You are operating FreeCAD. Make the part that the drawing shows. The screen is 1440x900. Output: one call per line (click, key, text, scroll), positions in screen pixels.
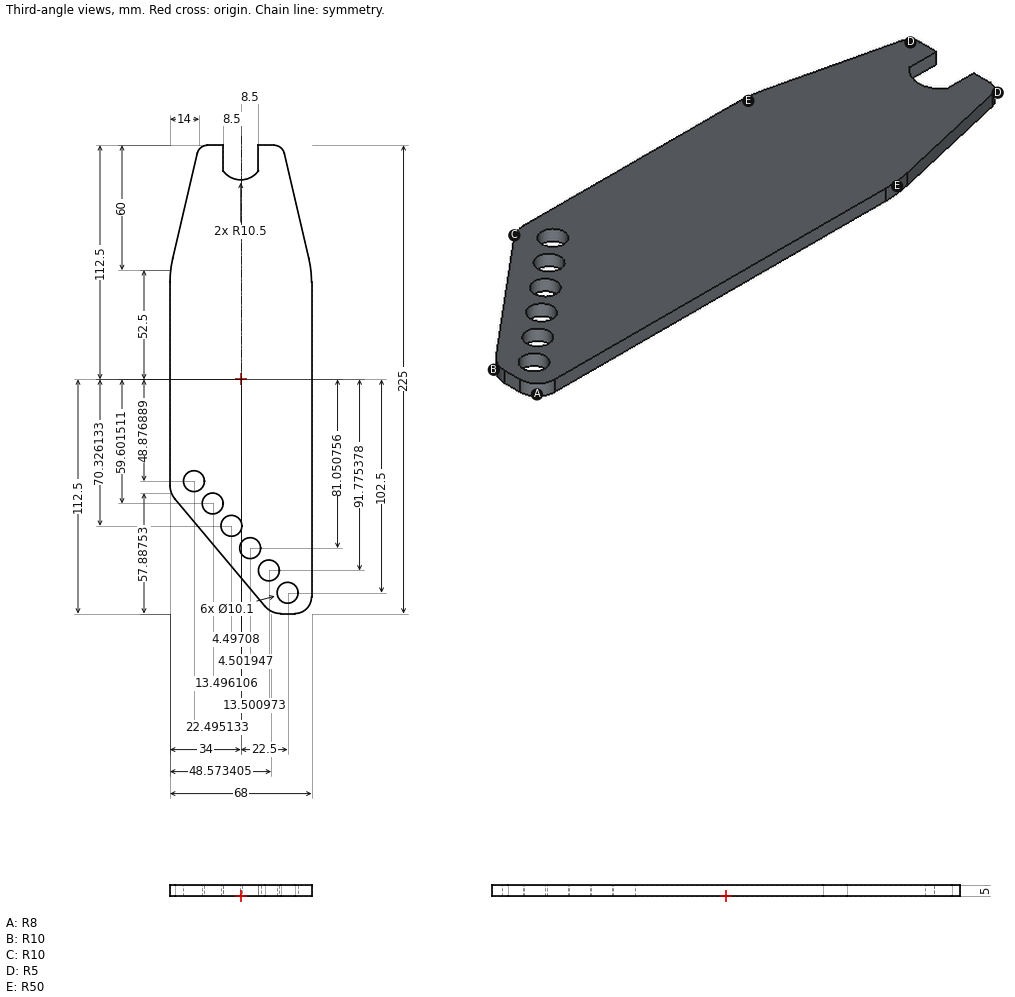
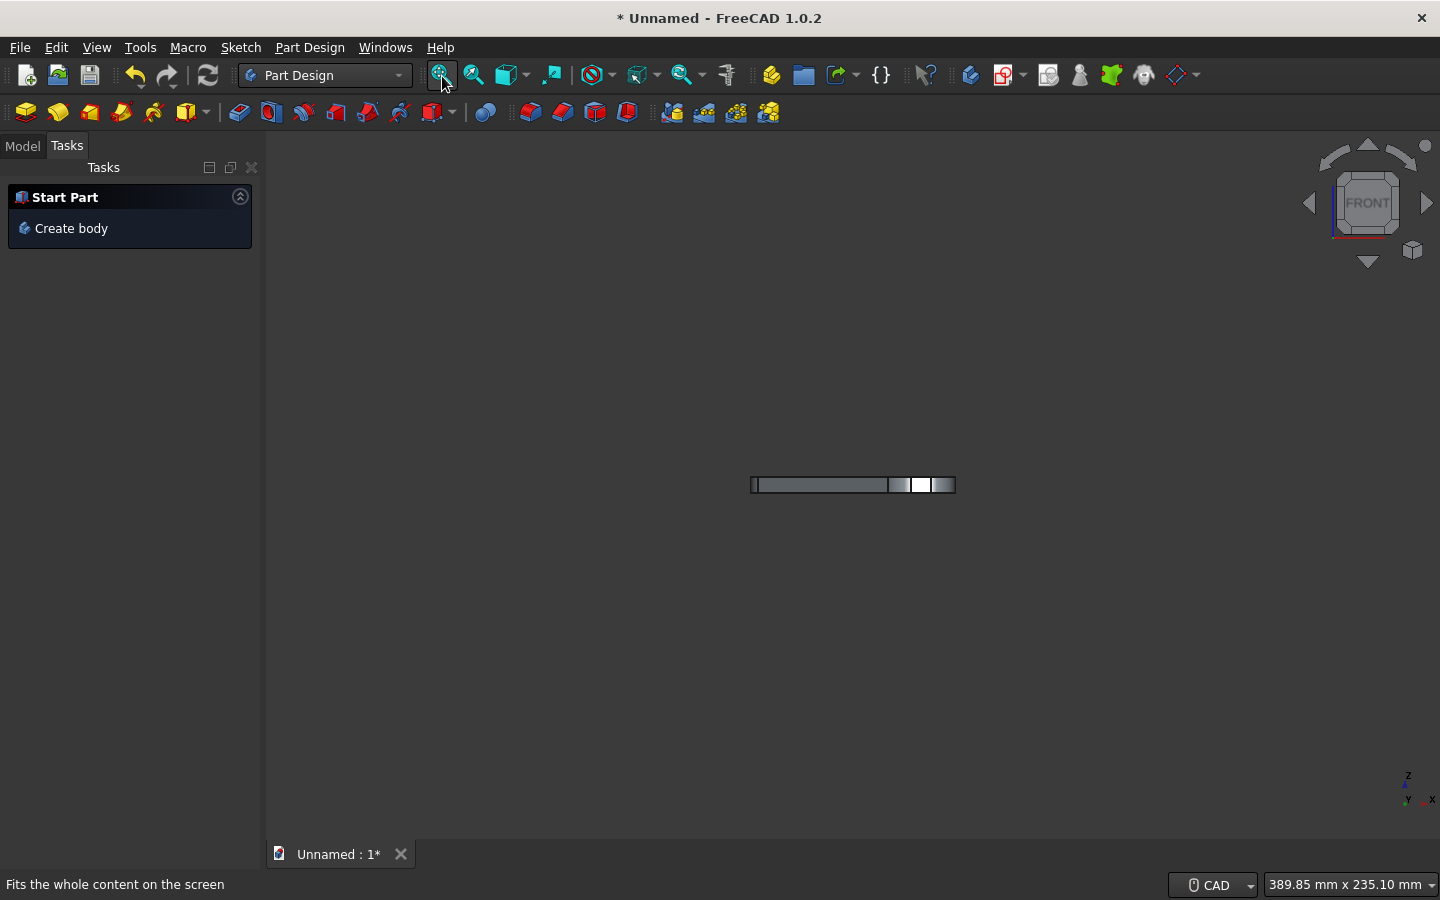
scroll(751, 484, up, 5)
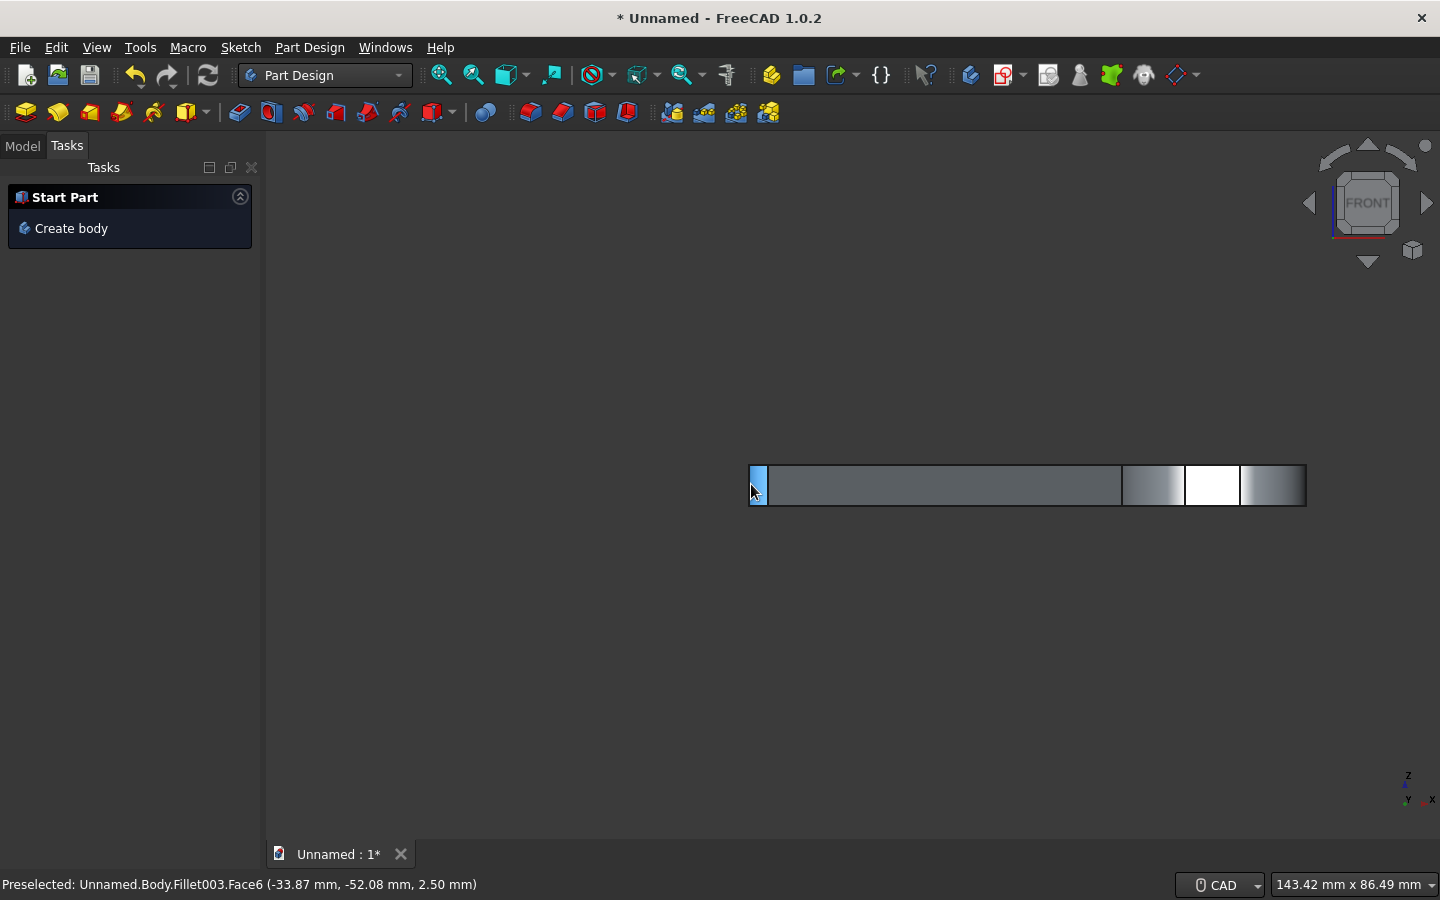
key(v)
key(f)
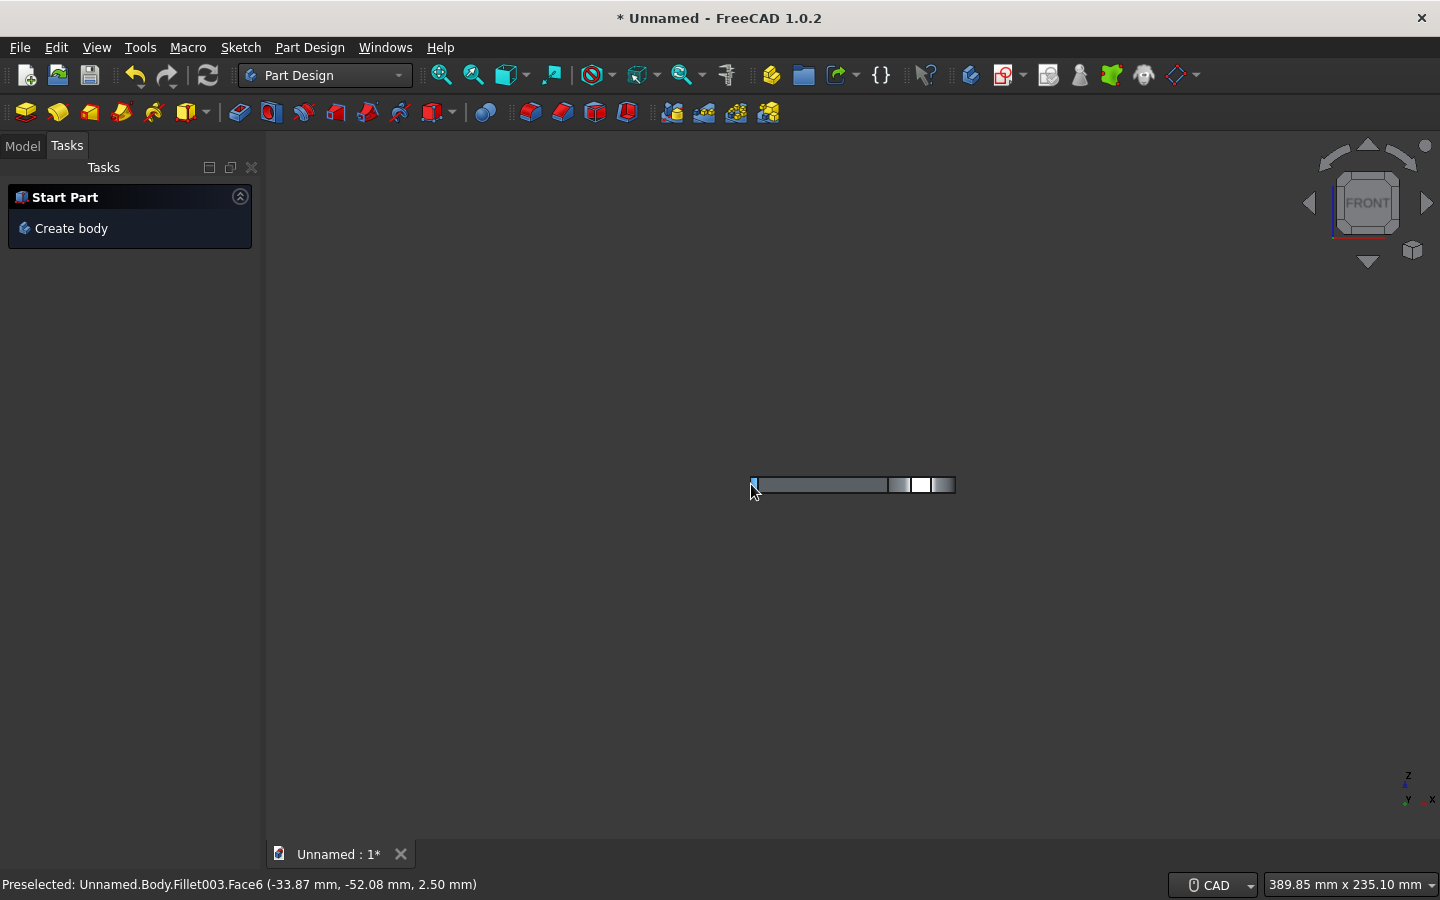
key(3)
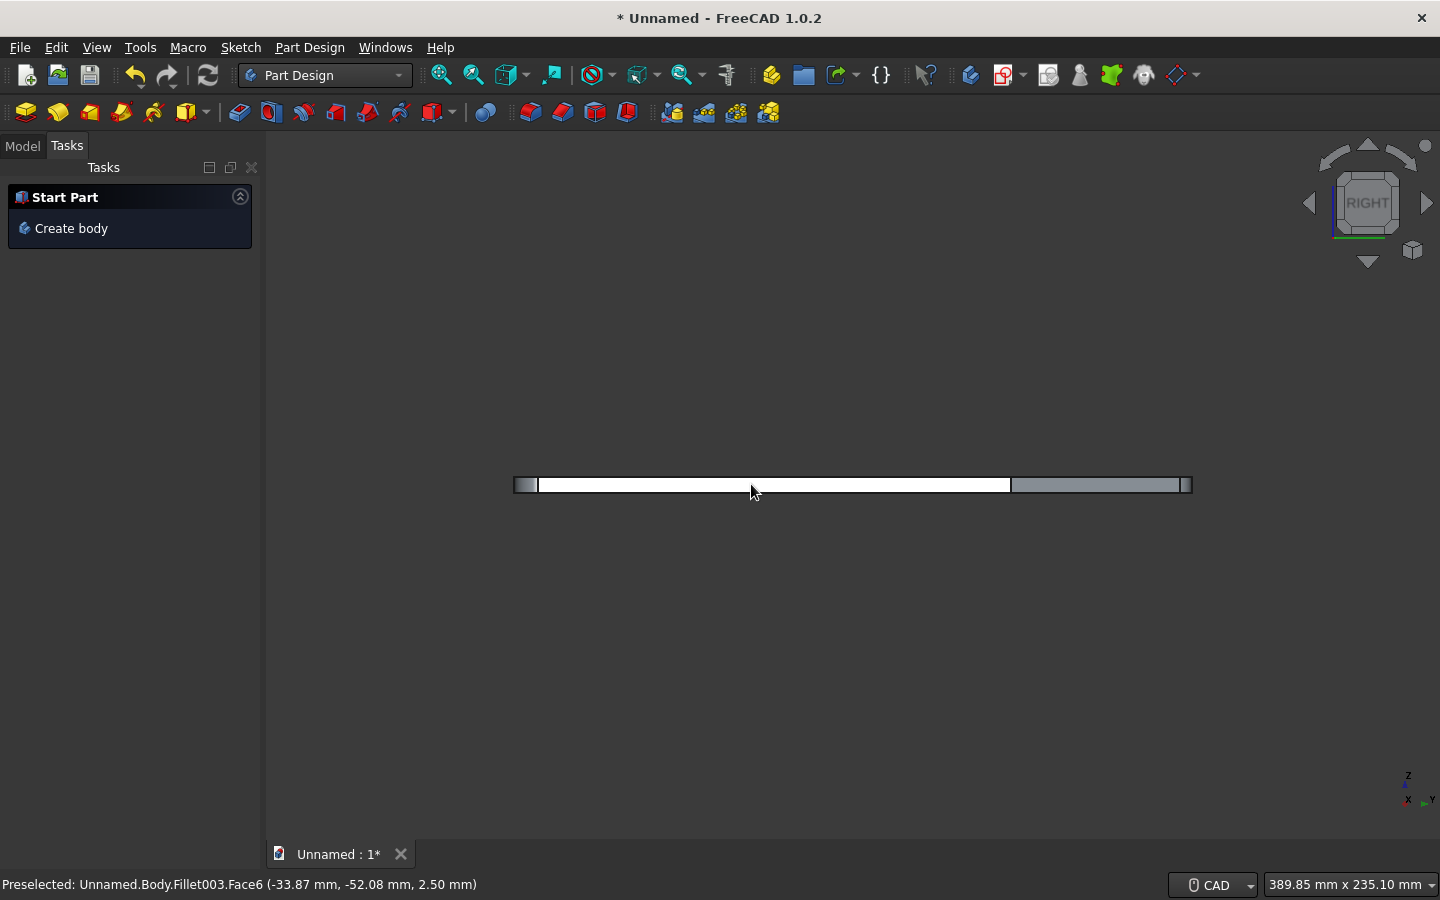
click(1011, 484)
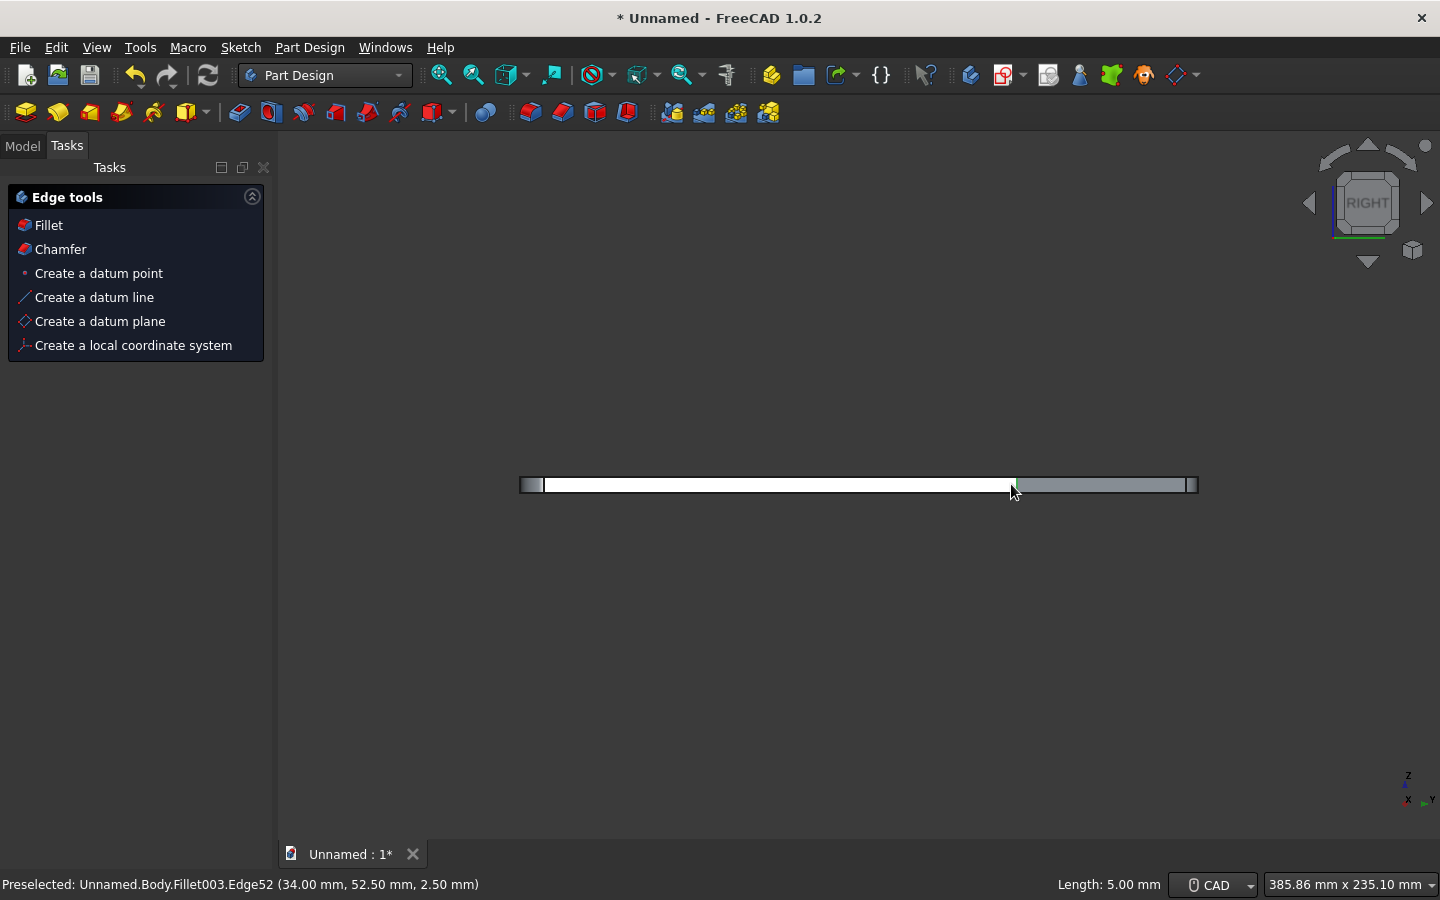
scroll(1017, 484, up, 5)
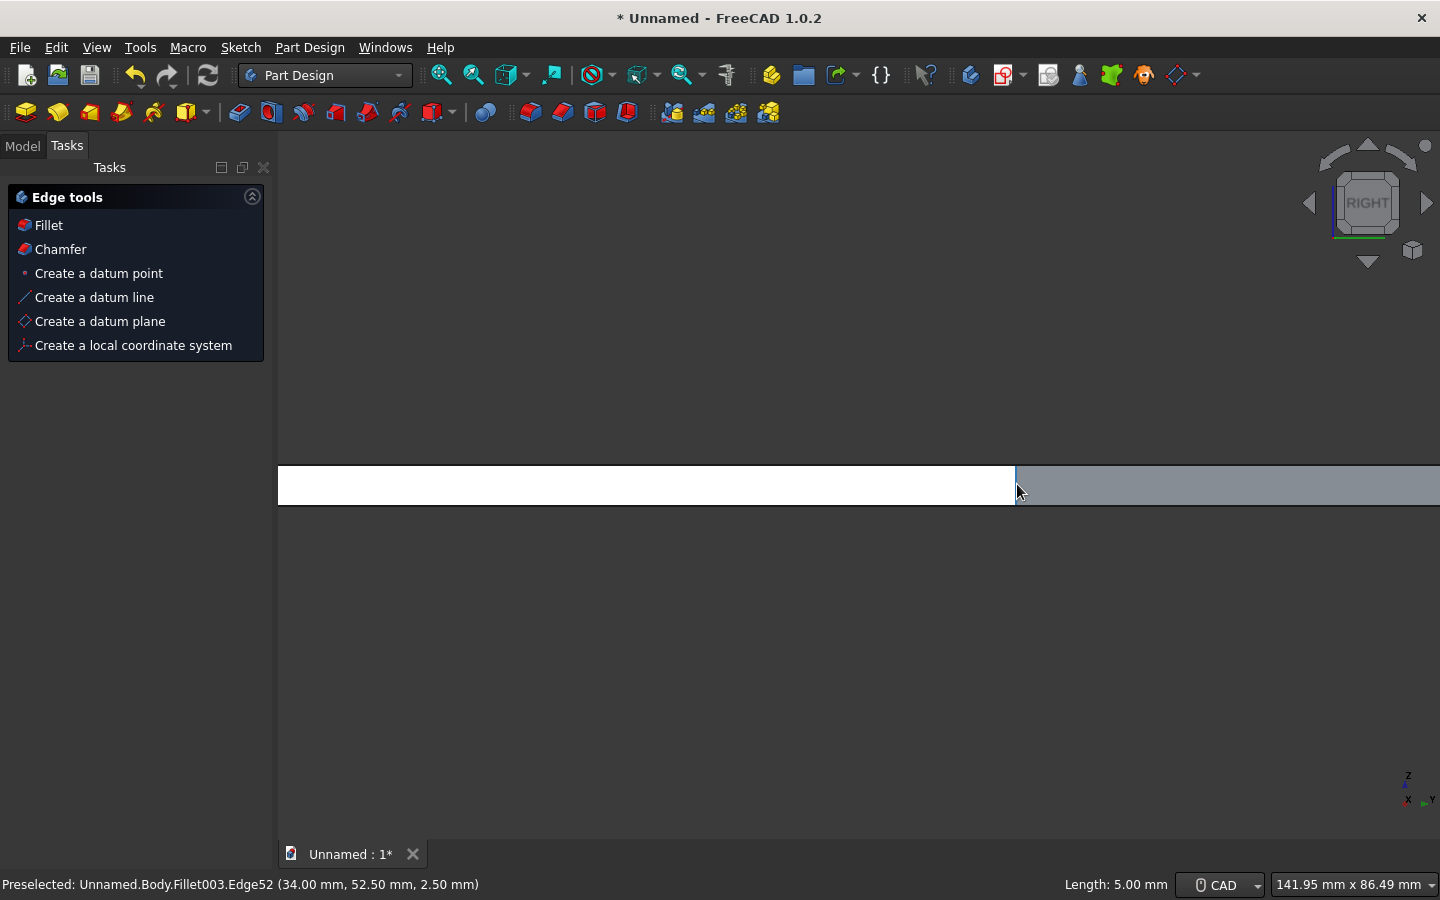
key(v)
key(f)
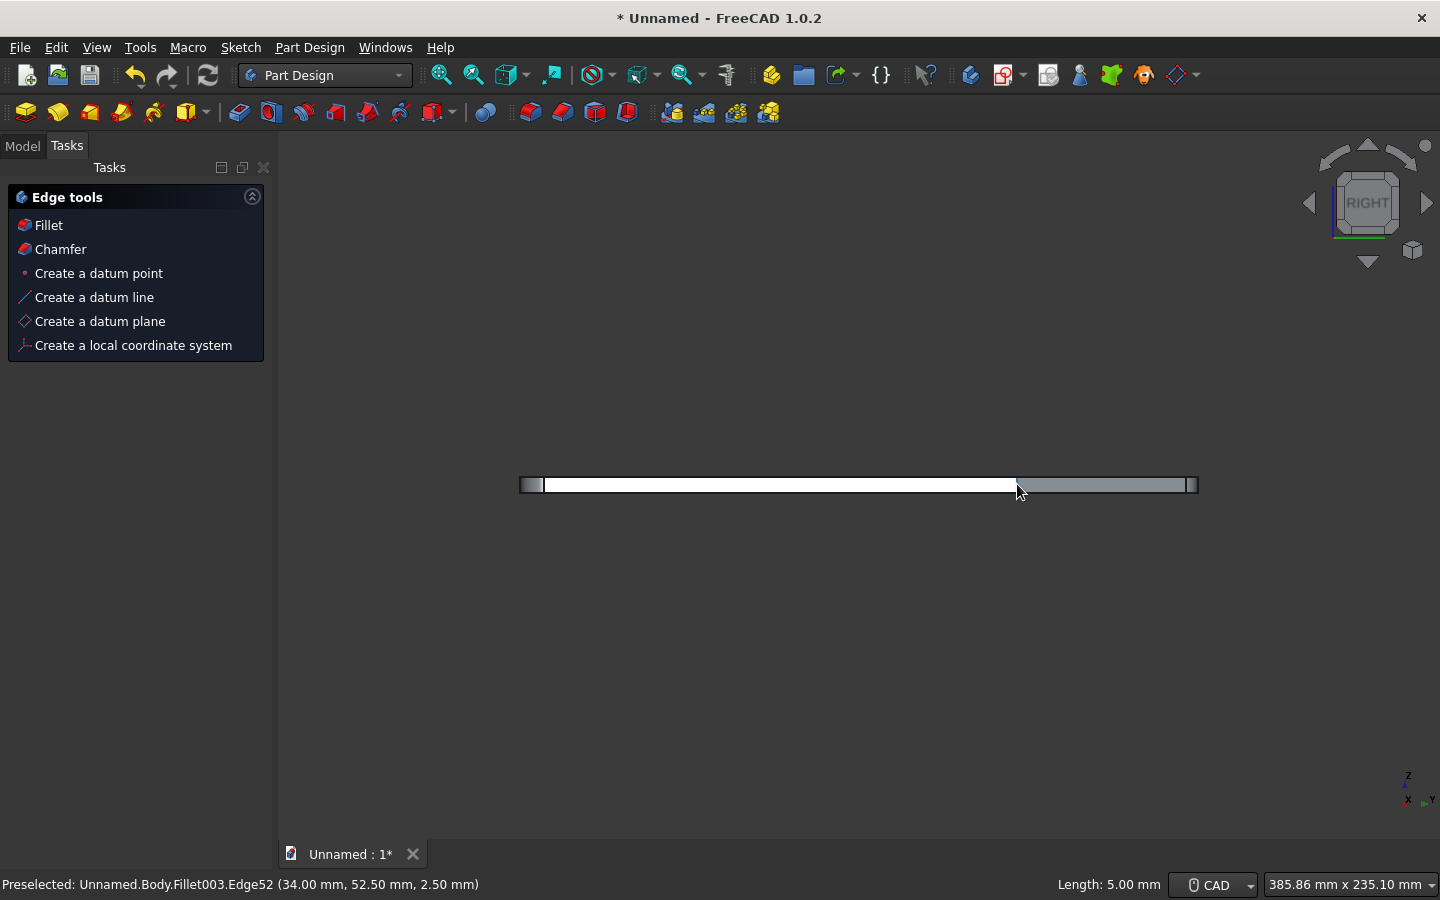
key(5)